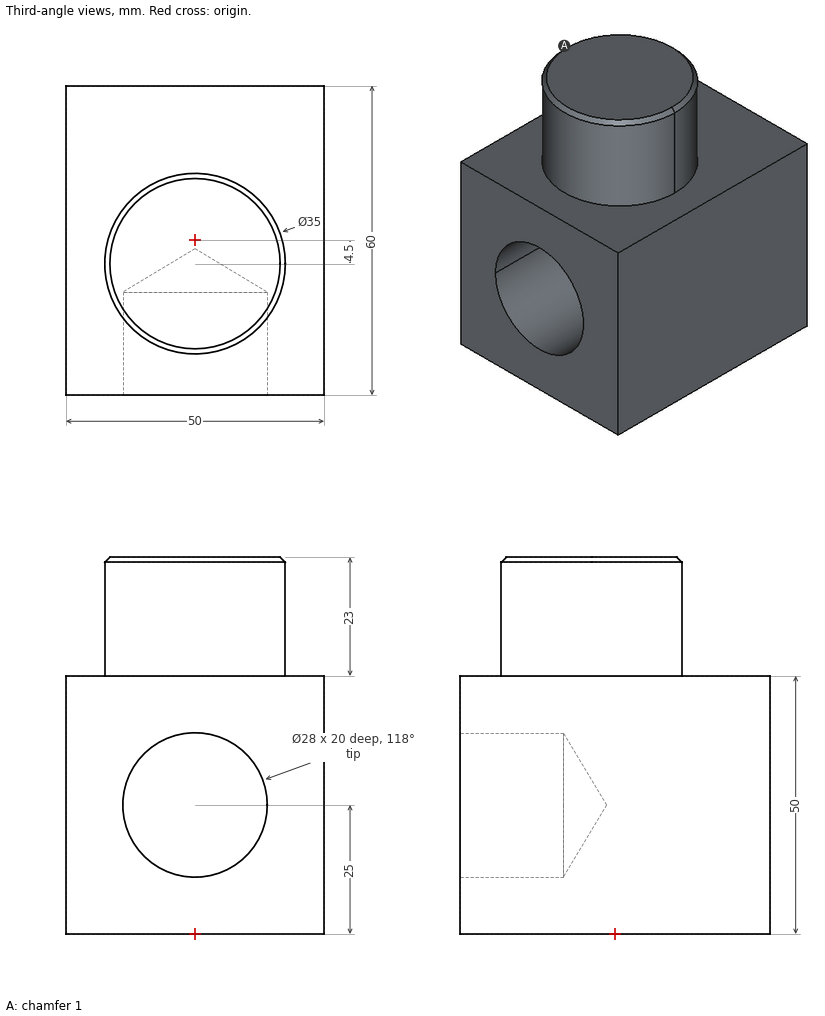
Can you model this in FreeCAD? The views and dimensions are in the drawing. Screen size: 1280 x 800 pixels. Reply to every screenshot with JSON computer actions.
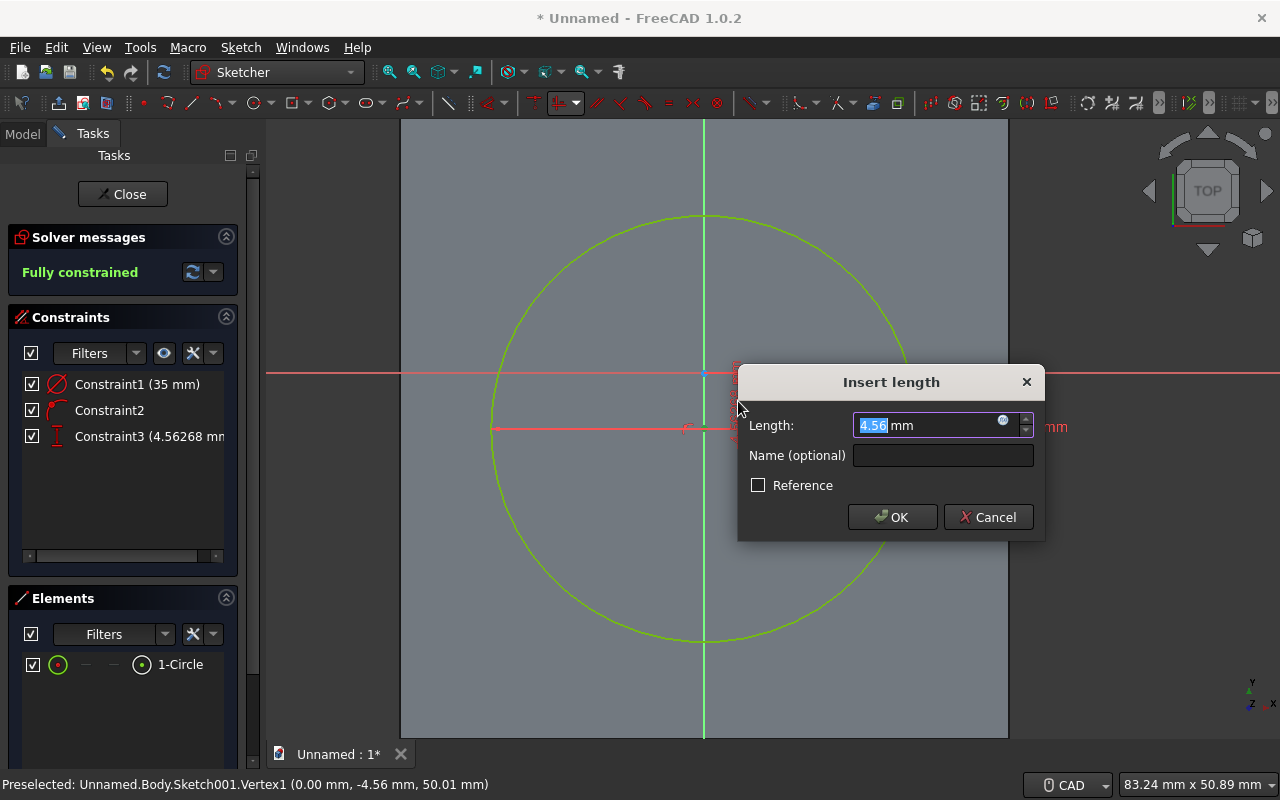
{"action": "type", "text": "4.5"}
{"action": "key", "text": "Return"}
{"action": "key", "text": "Escape"}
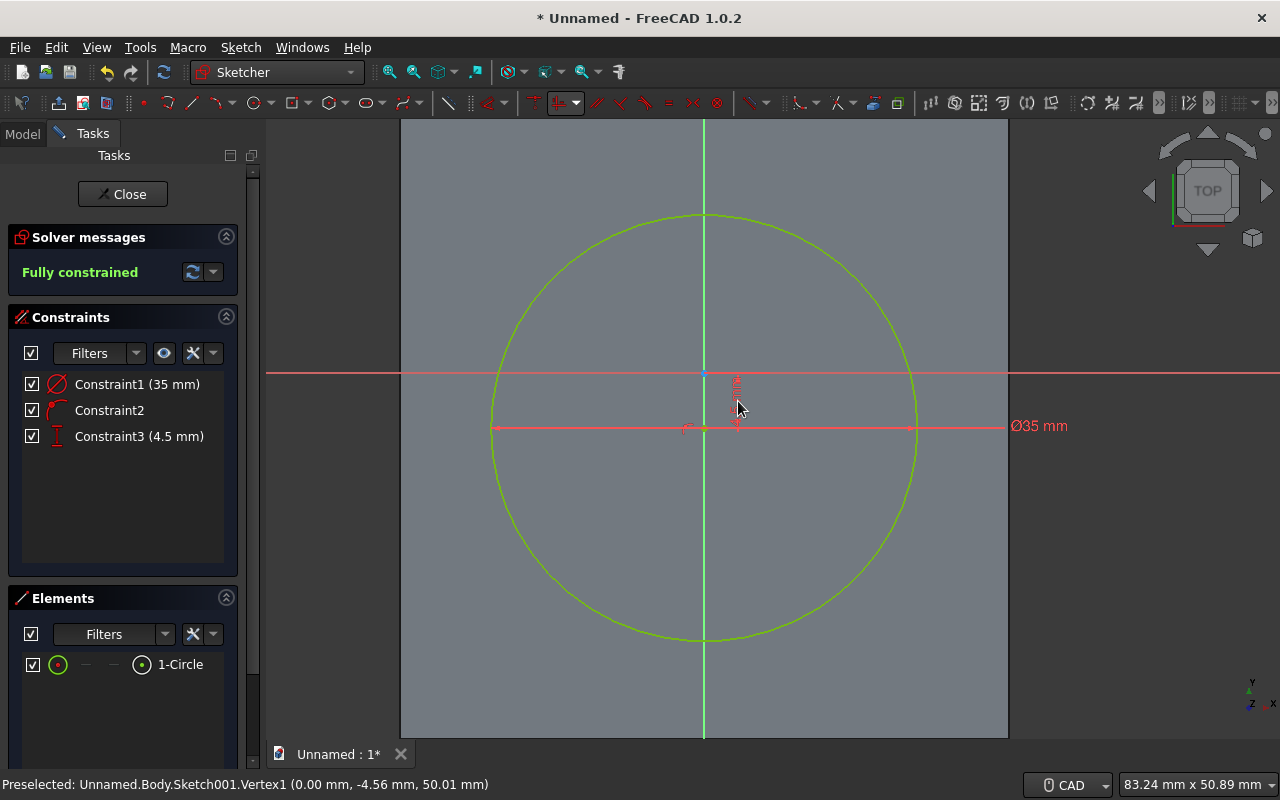
{"action": "left_click", "coordinate": [123, 194]}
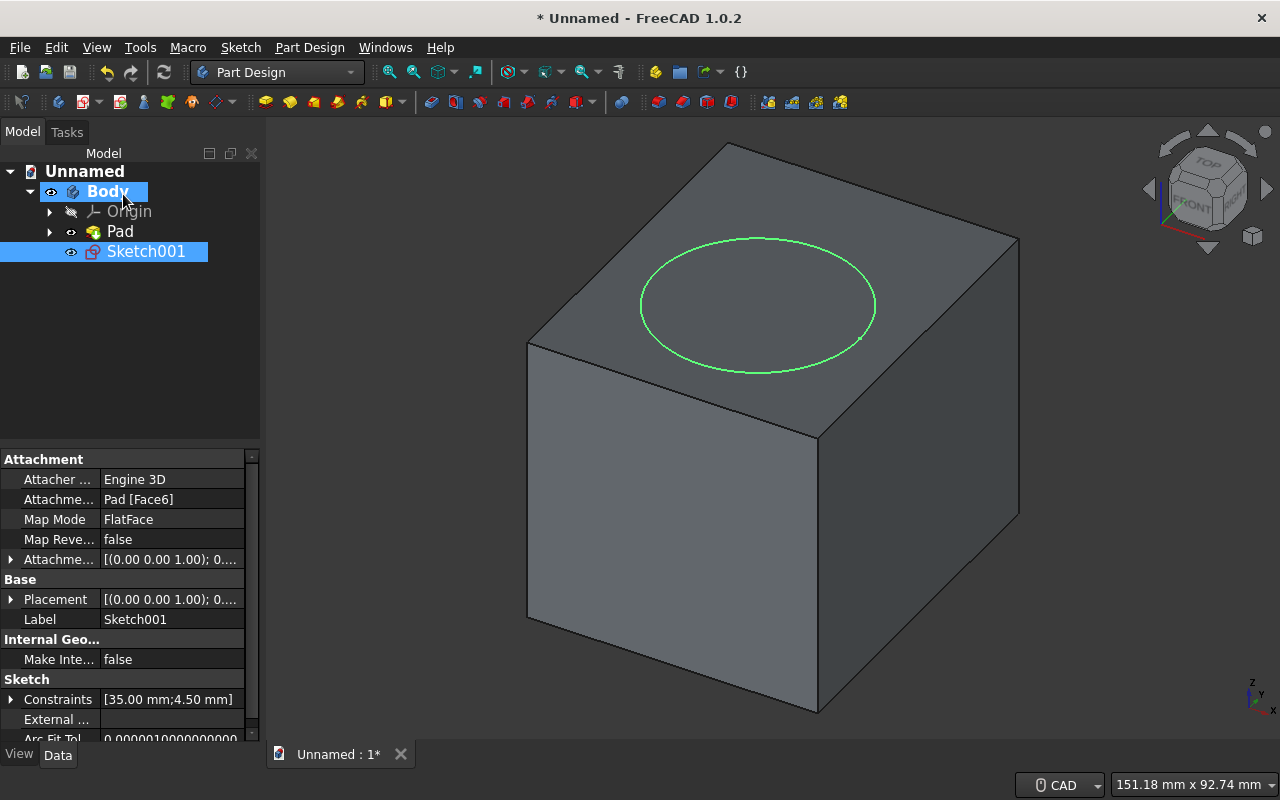
{"action": "left_click", "coordinate": [266, 102]}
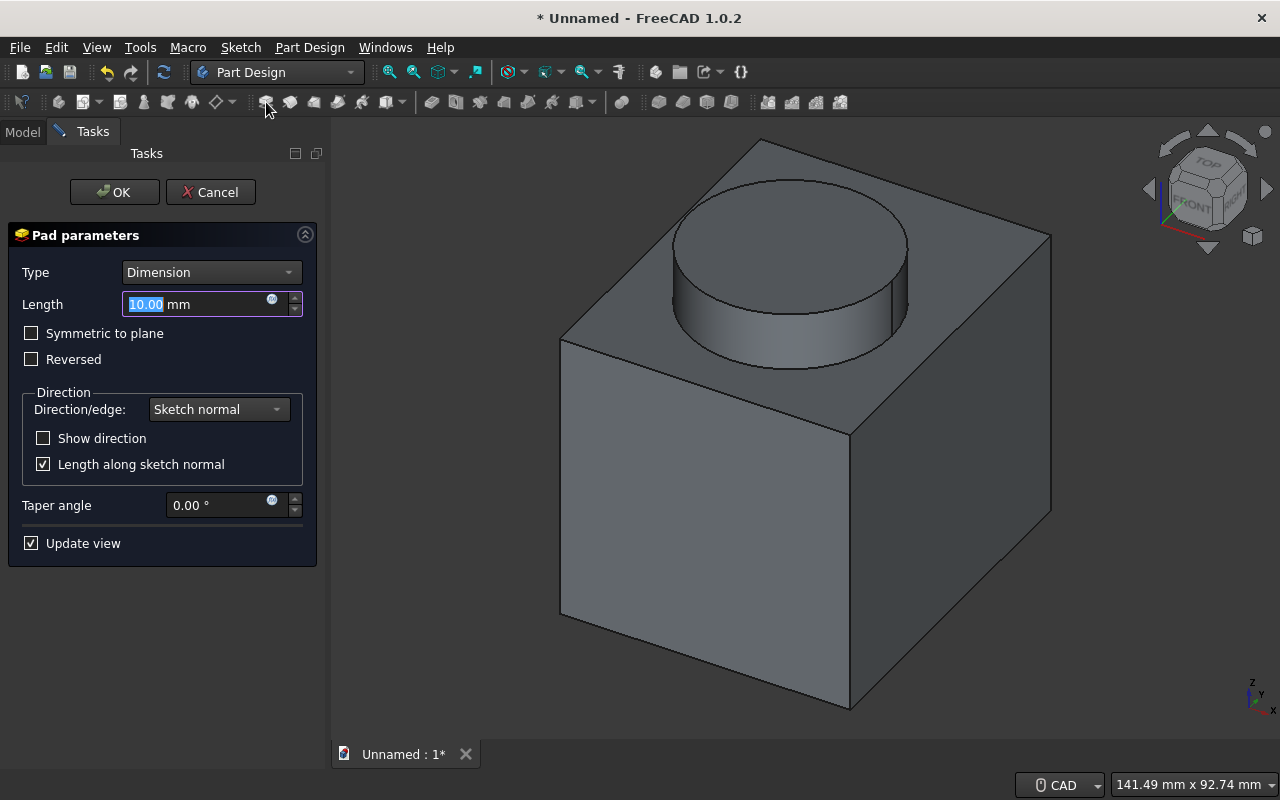
{"action": "type", "text": "23"}
{"action": "key", "text": "Tab"}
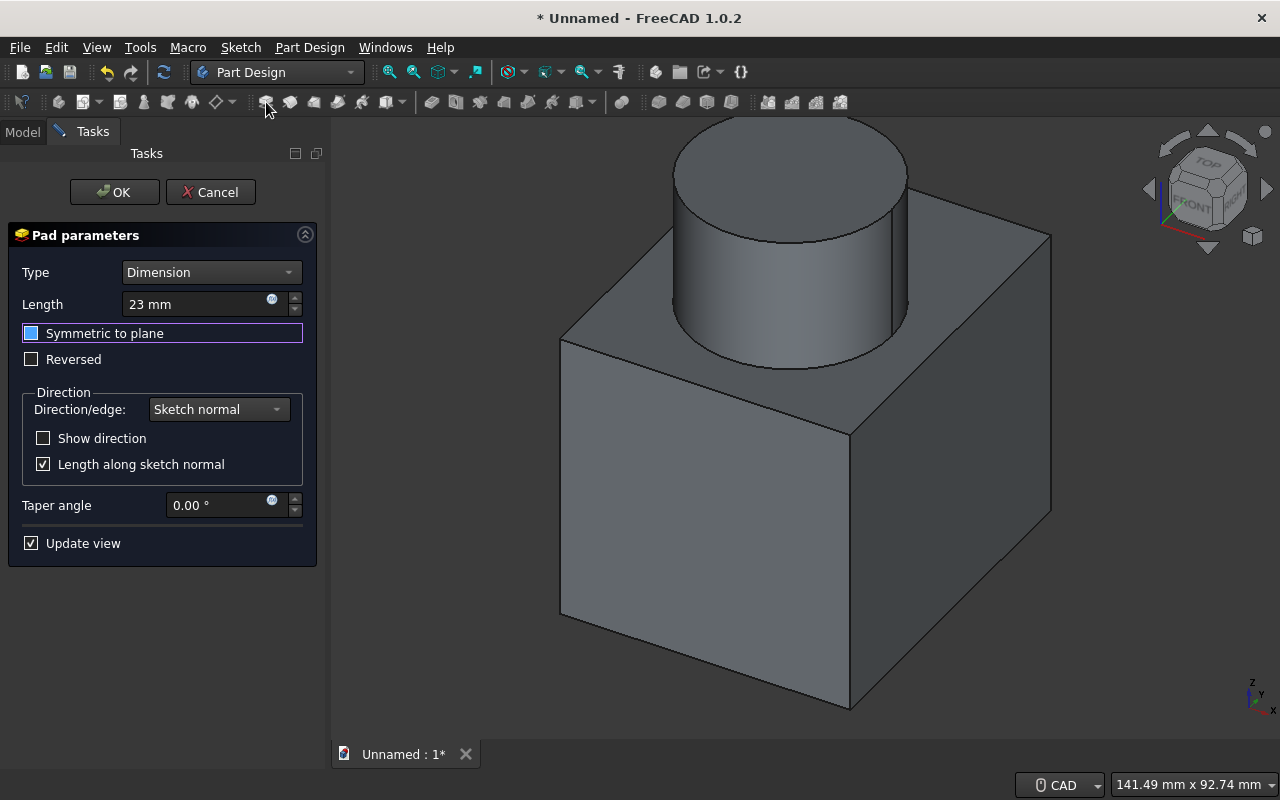
{"action": "left_click", "coordinate": [115, 192]}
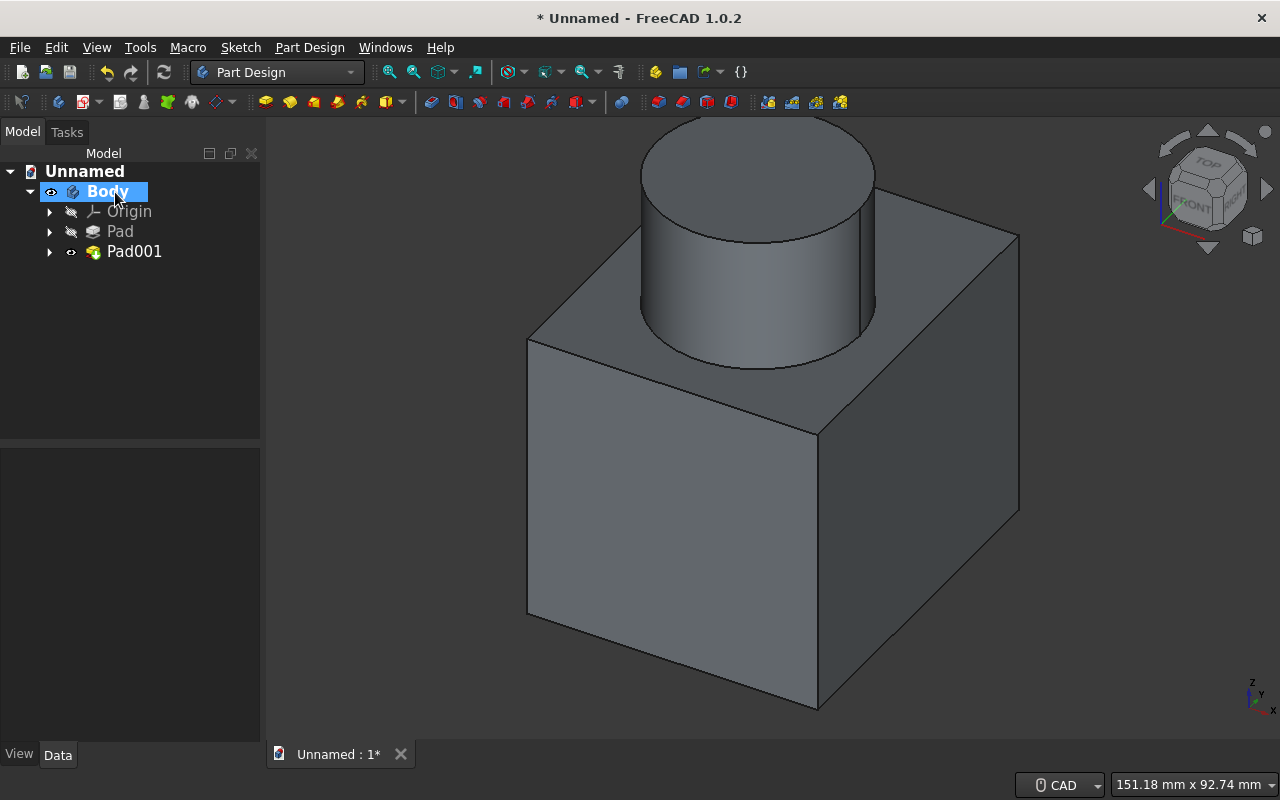
{"action": "left_click", "coordinate": [390, 72]}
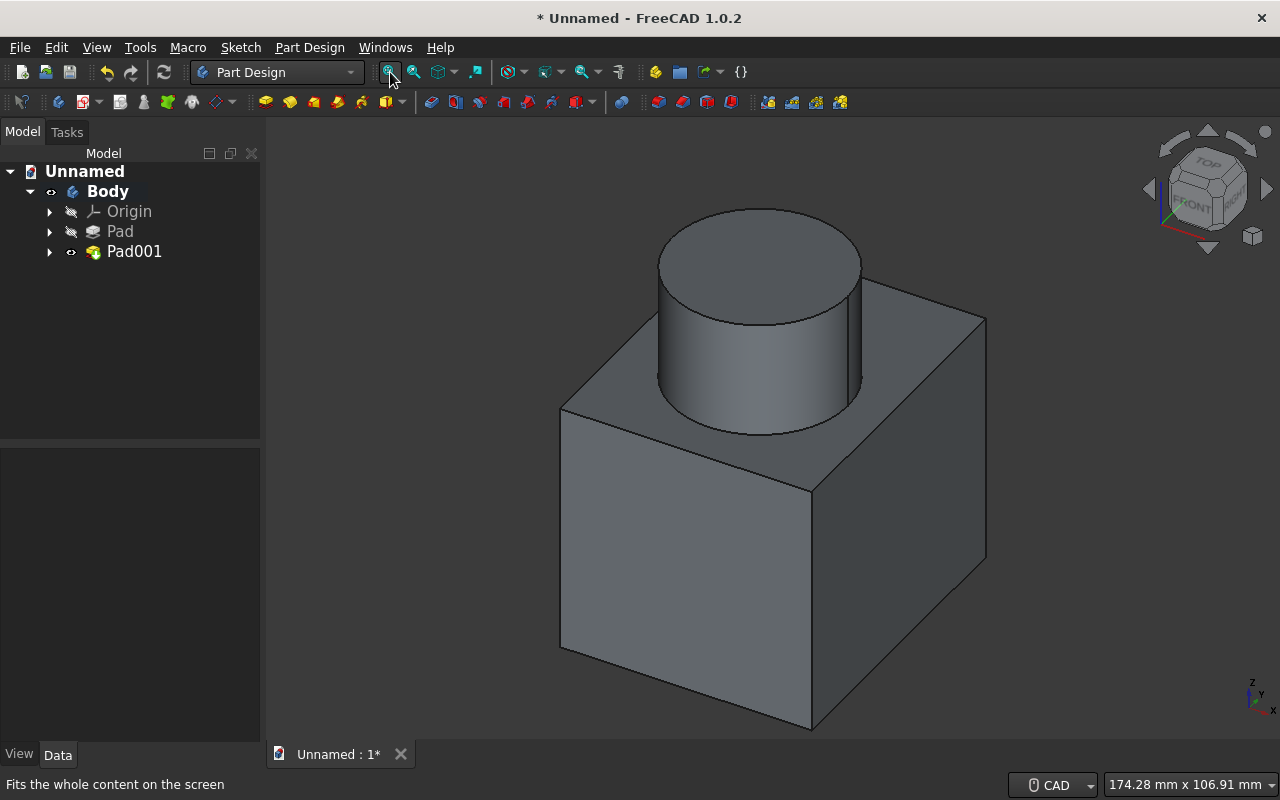
{"action": "left_click", "coordinate": [686, 569]}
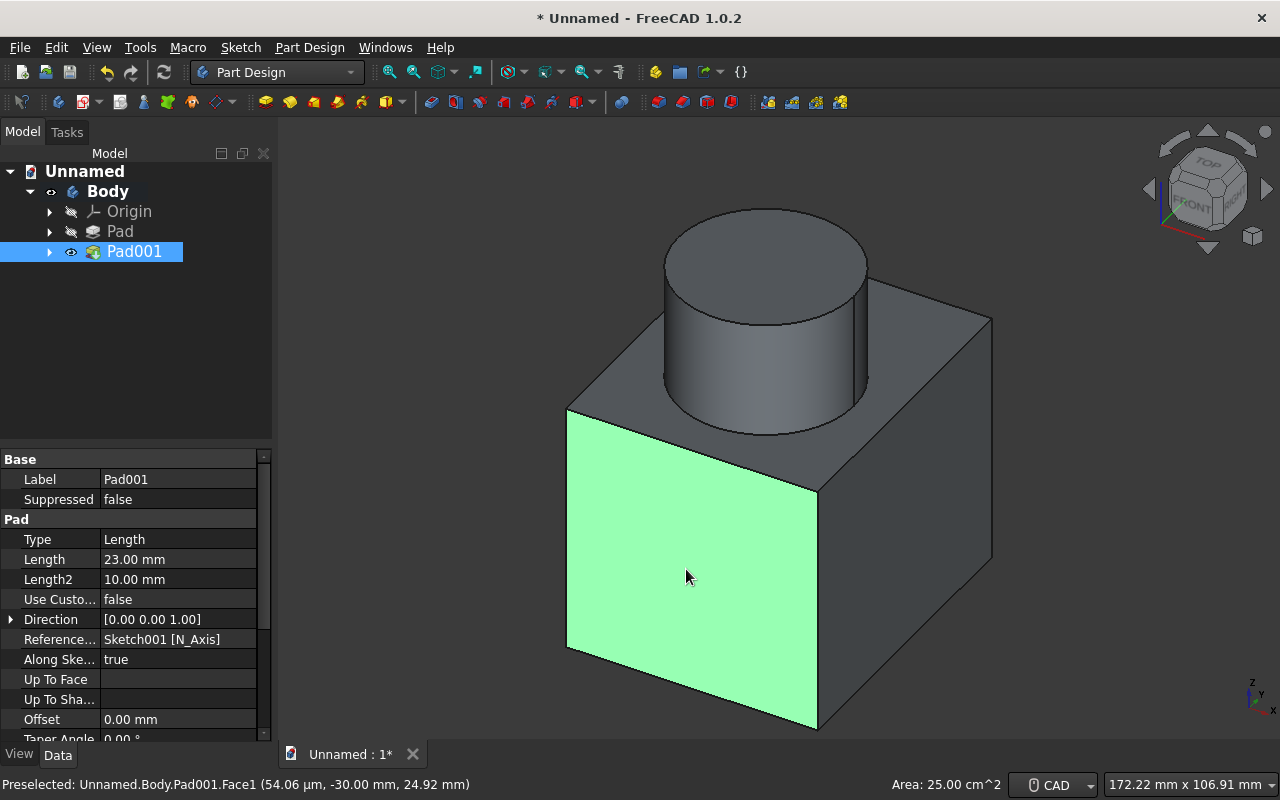
{"action": "left_click", "coordinate": [84, 102]}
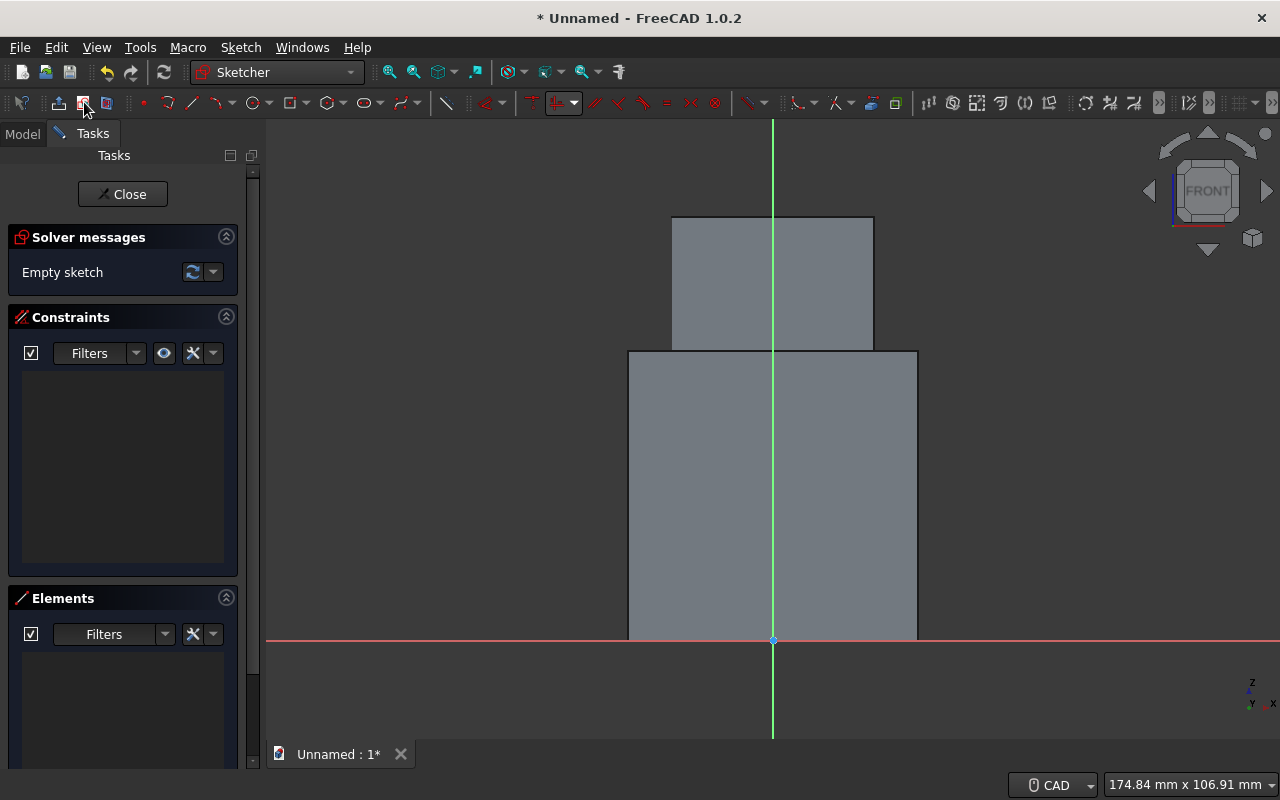
{"action": "scroll", "coordinate": [856, 648], "scroll_direction": "up", "scroll_amount": 3}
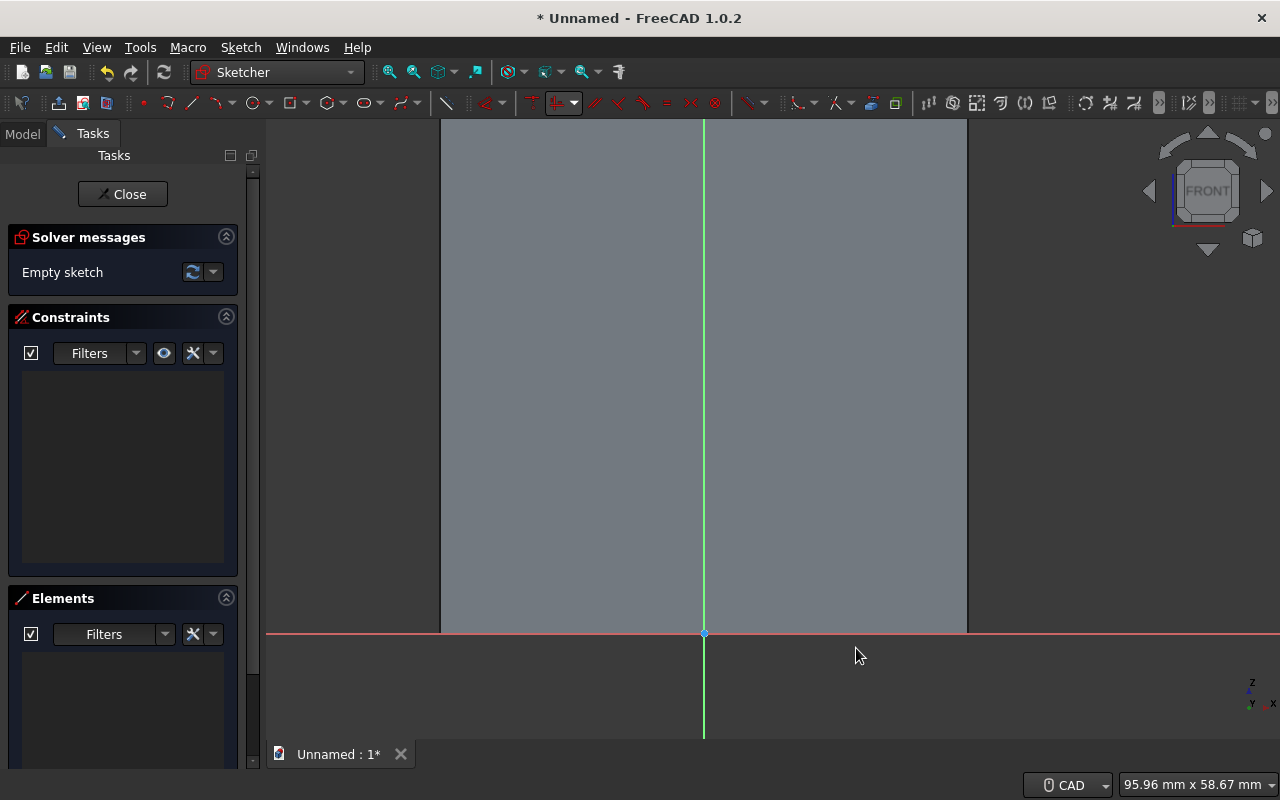
{"action": "left_click", "coordinate": [254, 104]}